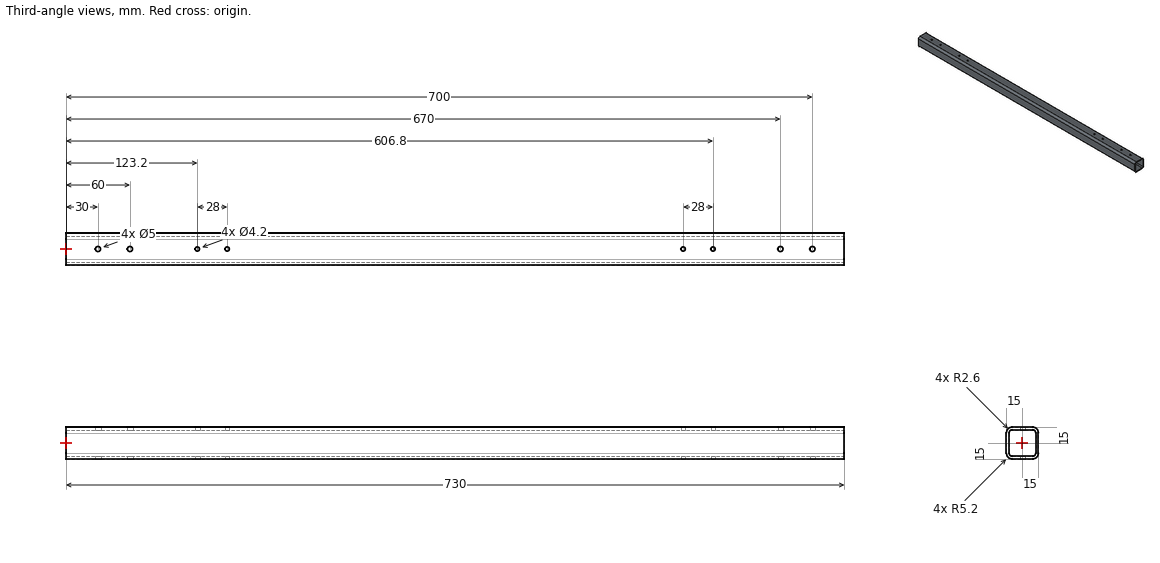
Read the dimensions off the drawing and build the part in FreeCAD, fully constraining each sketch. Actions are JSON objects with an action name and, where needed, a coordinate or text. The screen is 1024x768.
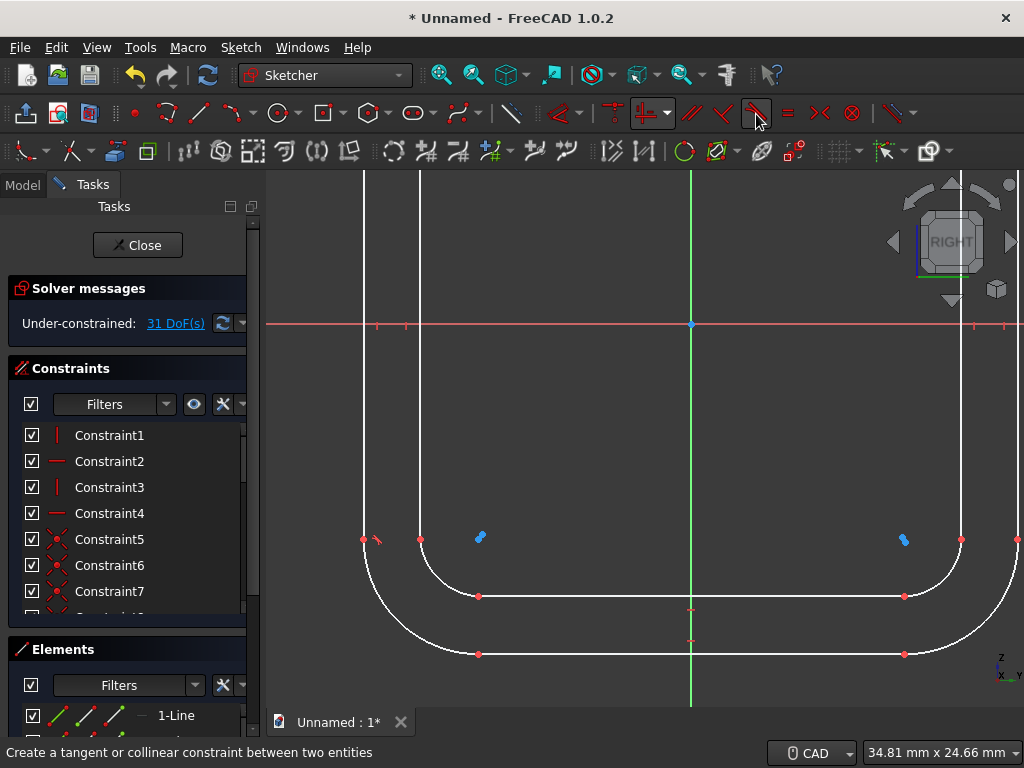
{"action": "left_click", "coordinate": [364, 240]}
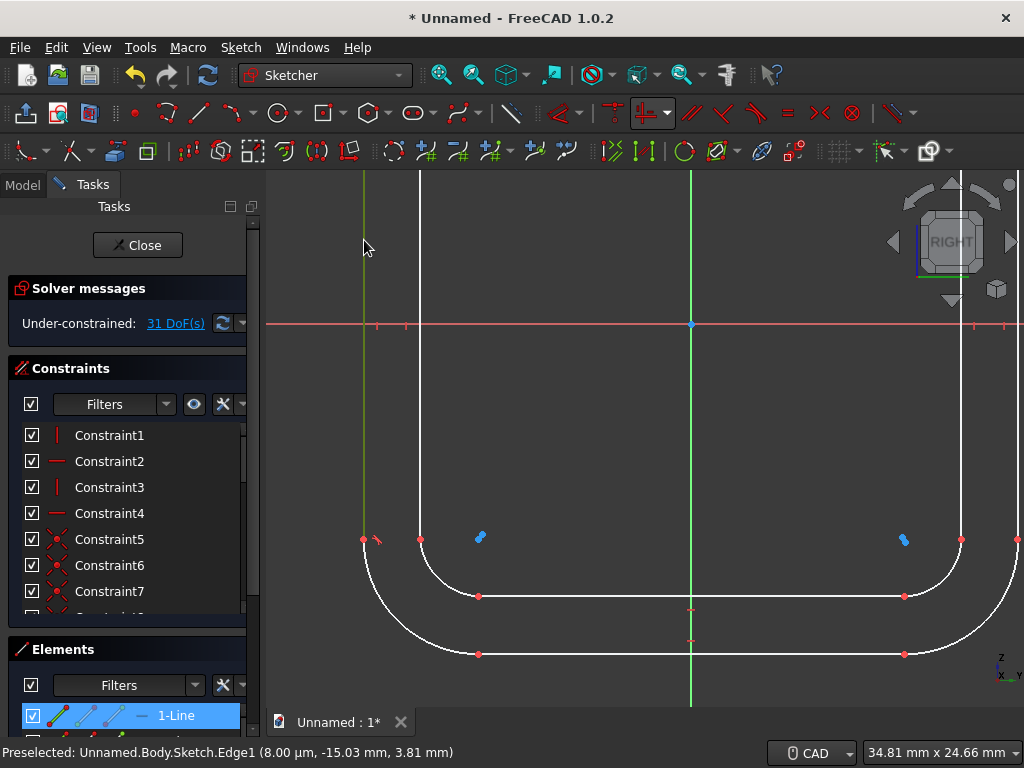
{"action": "scroll", "coordinate": [437, 578], "scroll_direction": "down", "scroll_amount": 3}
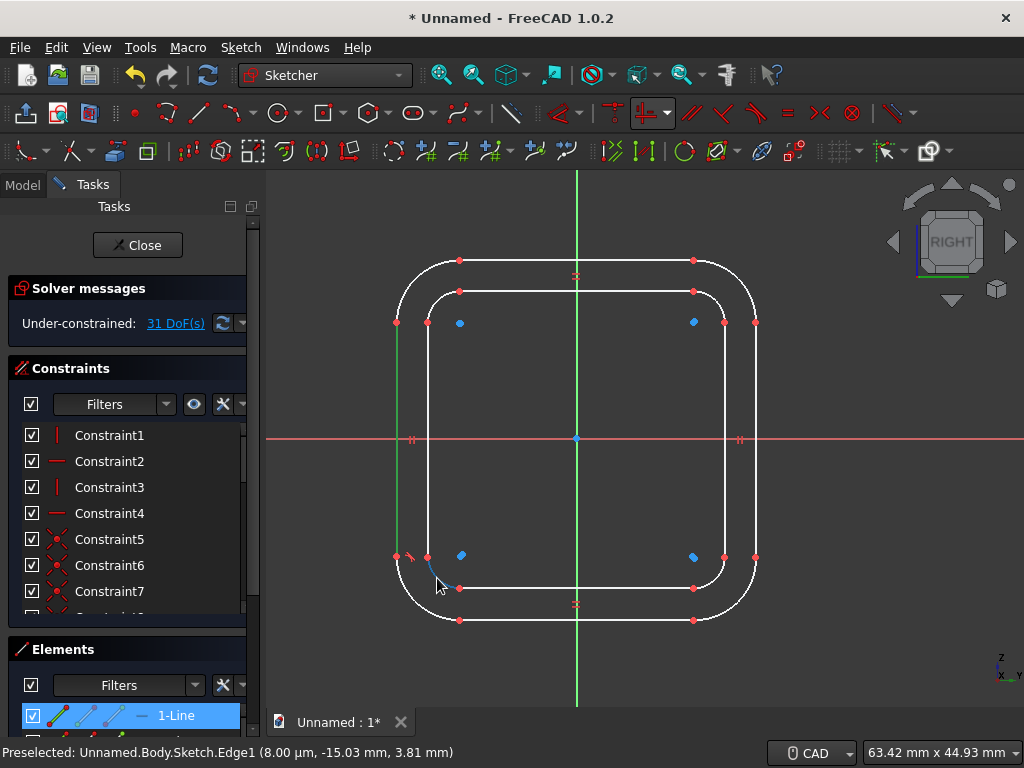
{"action": "left_click", "coordinate": [432, 267]}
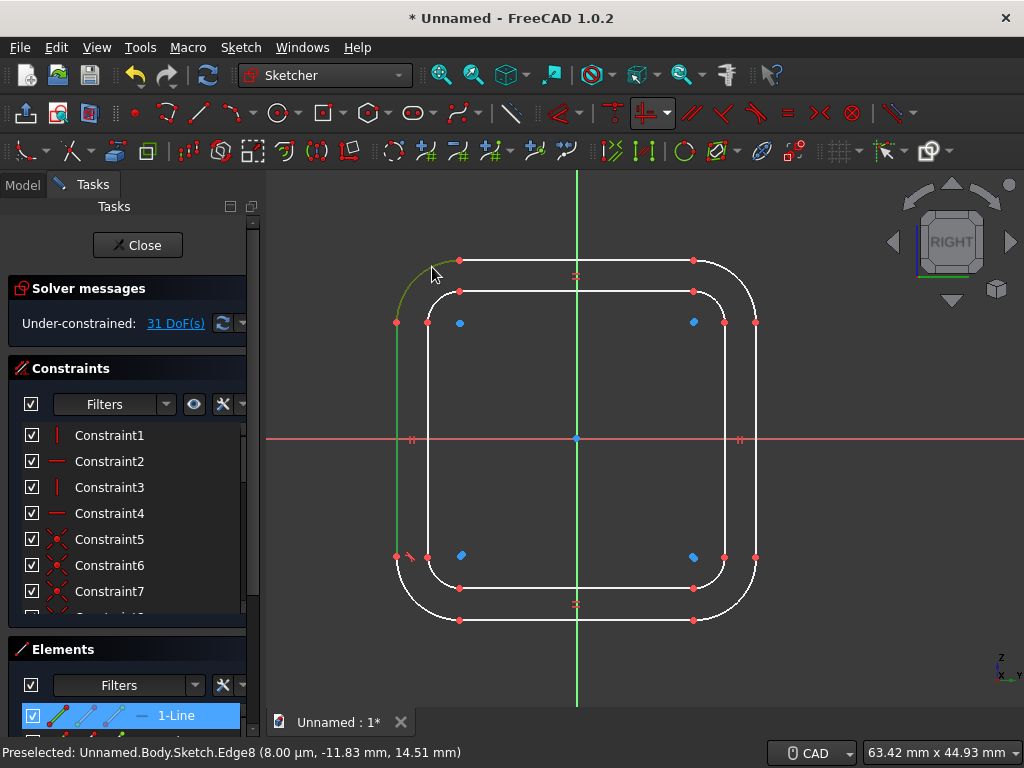
{"action": "left_click", "coordinate": [756, 114]}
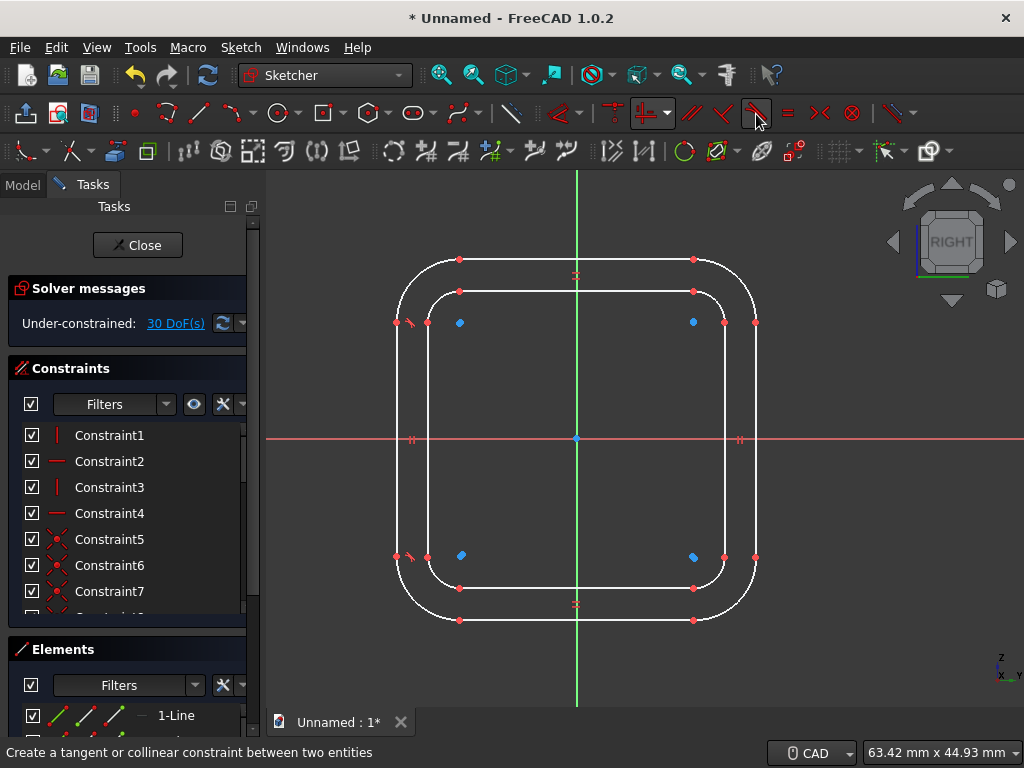
{"action": "left_click", "coordinate": [530, 620]}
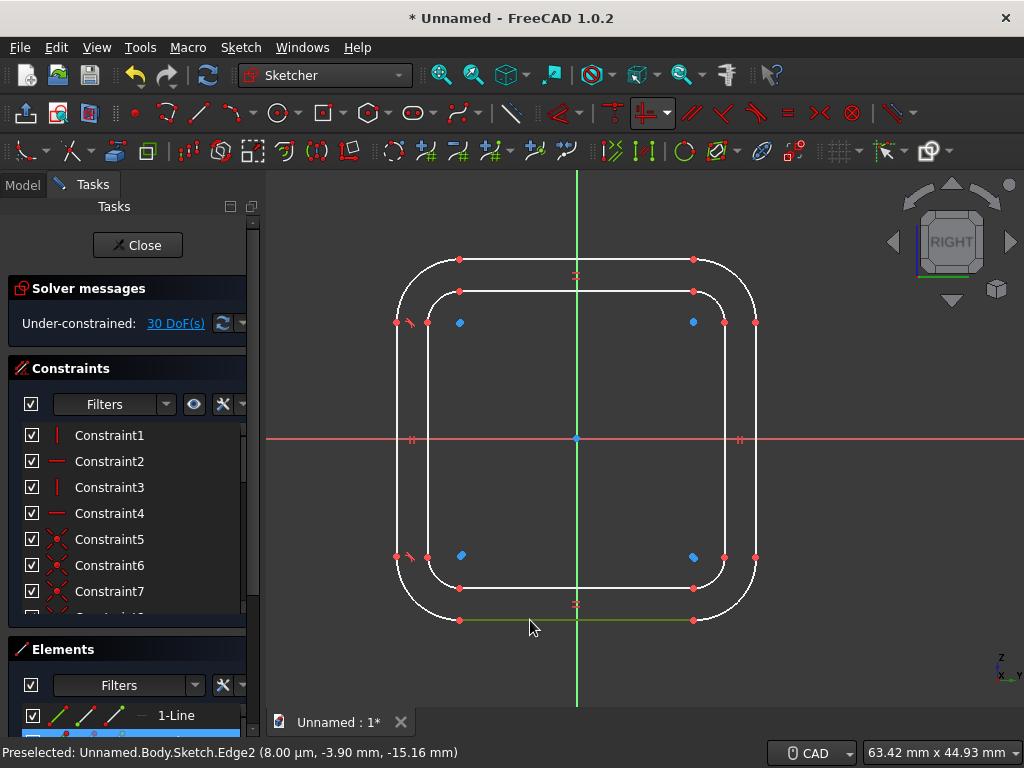
{"action": "left_click", "coordinate": [404, 586]}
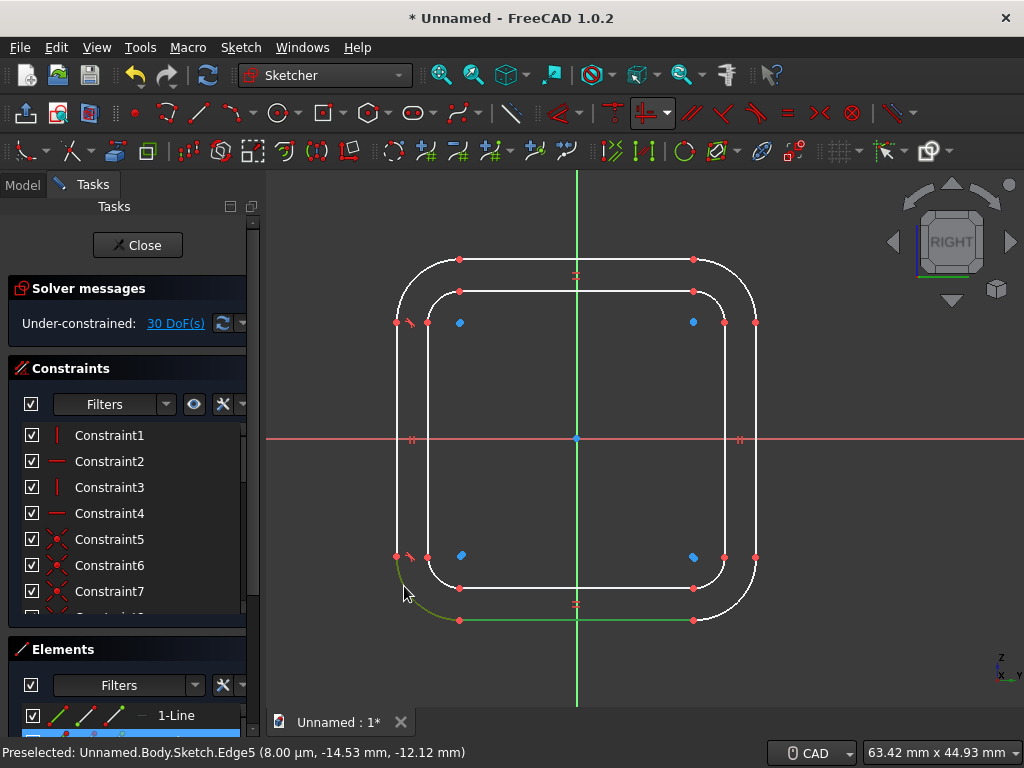
{"action": "left_click", "coordinate": [756, 114]}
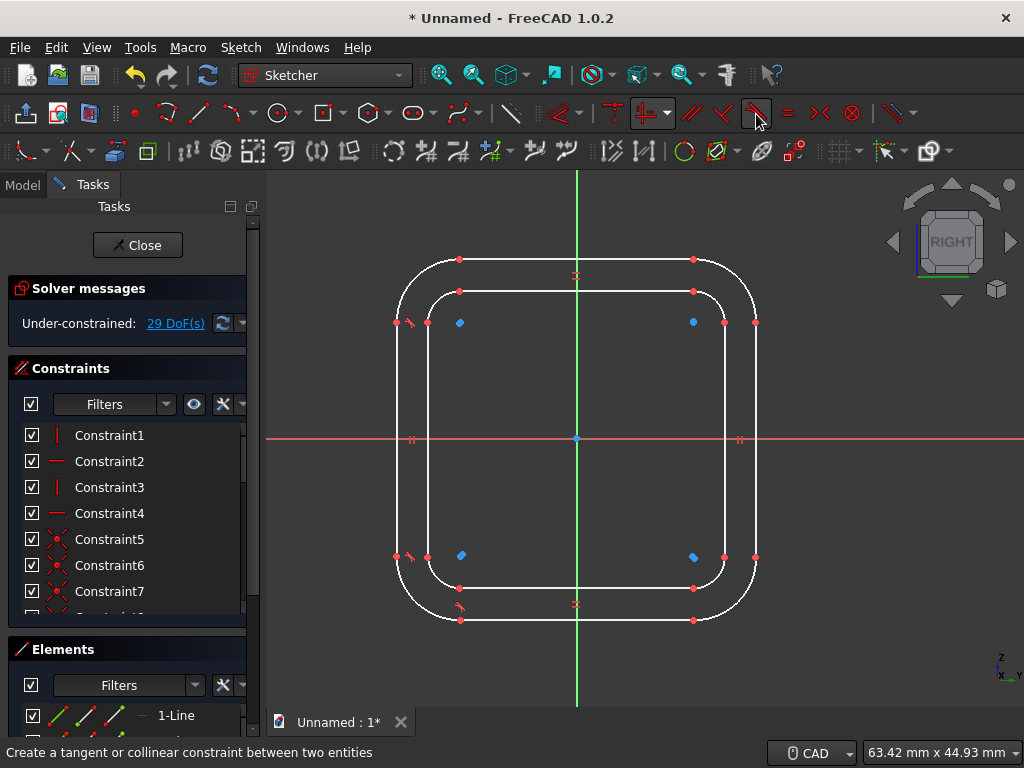
{"action": "left_click", "coordinate": [530, 620]}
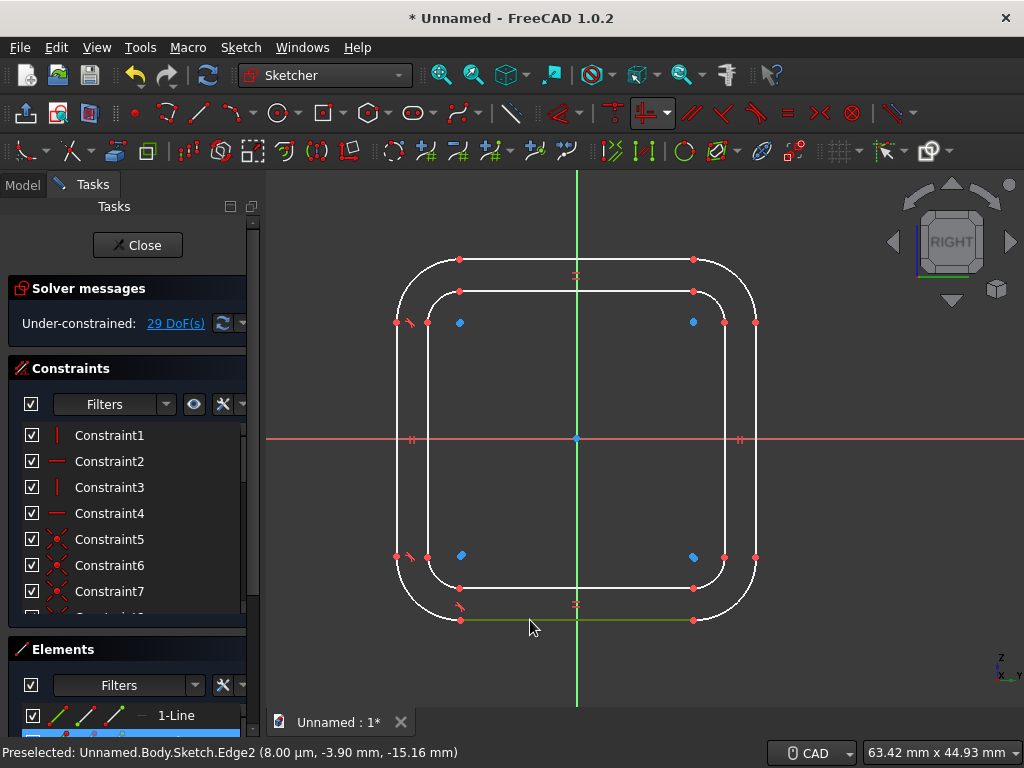
{"action": "left_click", "coordinate": [722, 613]}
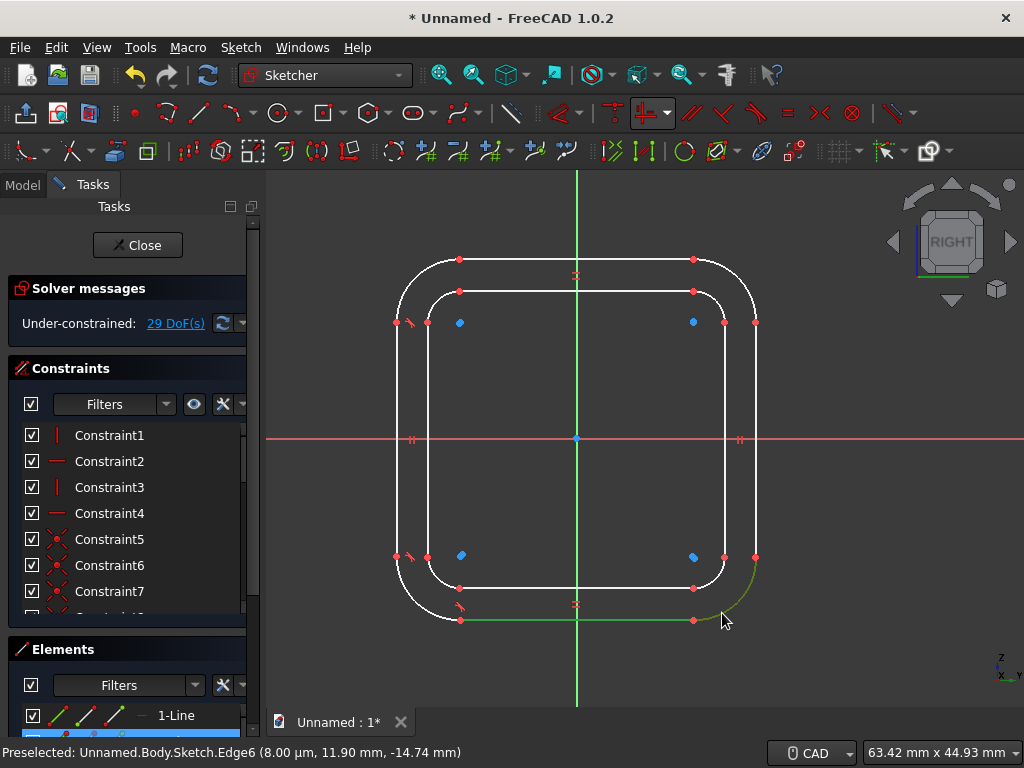
{"action": "left_click", "coordinate": [756, 114]}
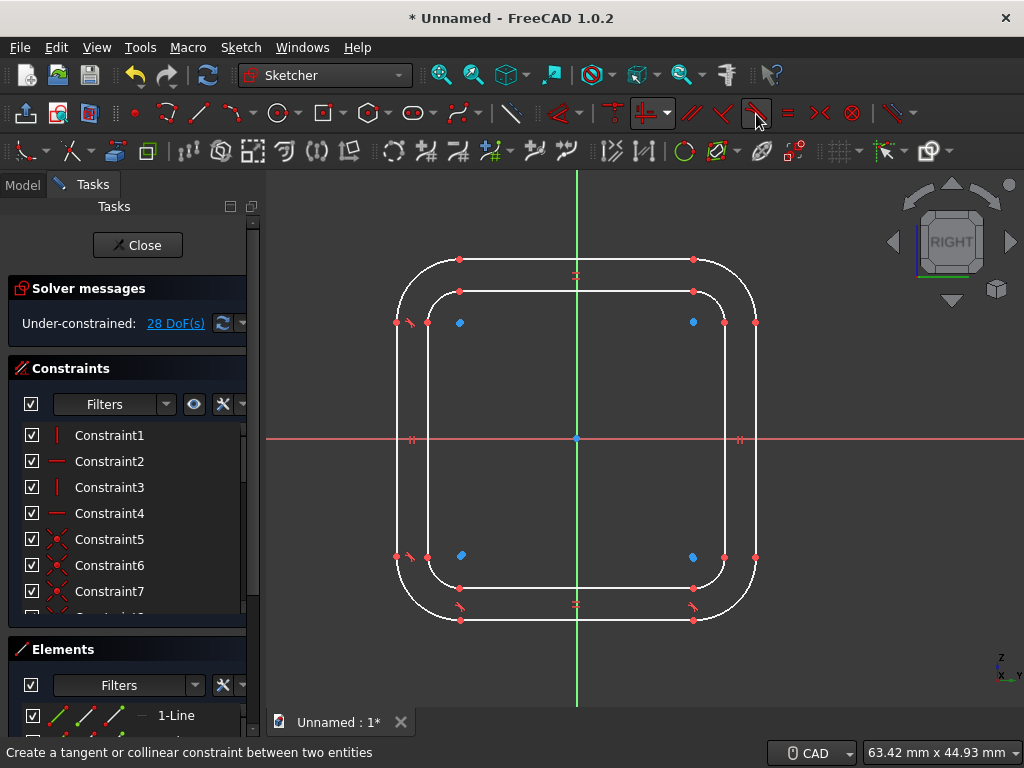
{"action": "left_click", "coordinate": [756, 487]}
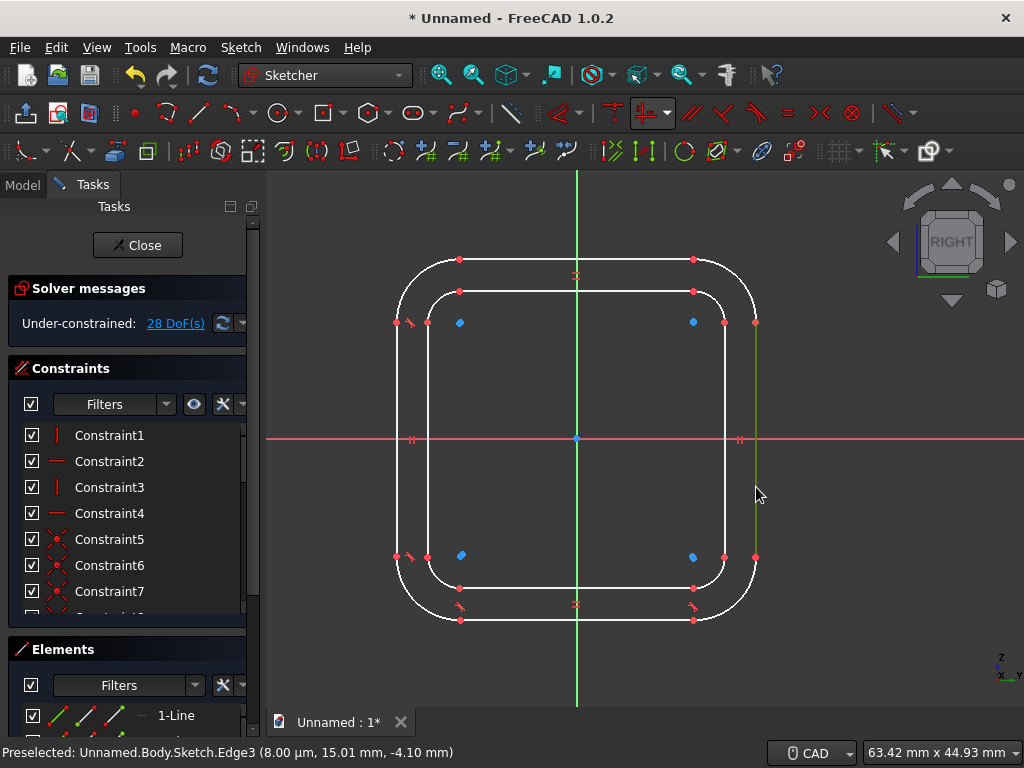
{"action": "left_click", "coordinate": [722, 613]}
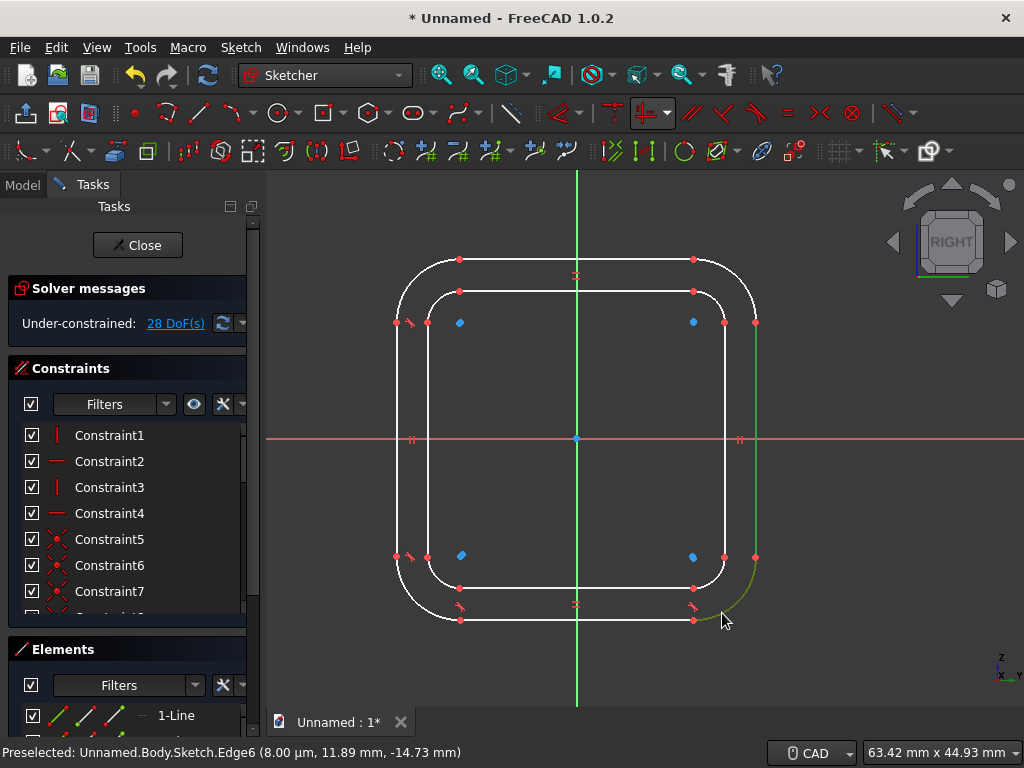
{"action": "left_click", "coordinate": [756, 114]}